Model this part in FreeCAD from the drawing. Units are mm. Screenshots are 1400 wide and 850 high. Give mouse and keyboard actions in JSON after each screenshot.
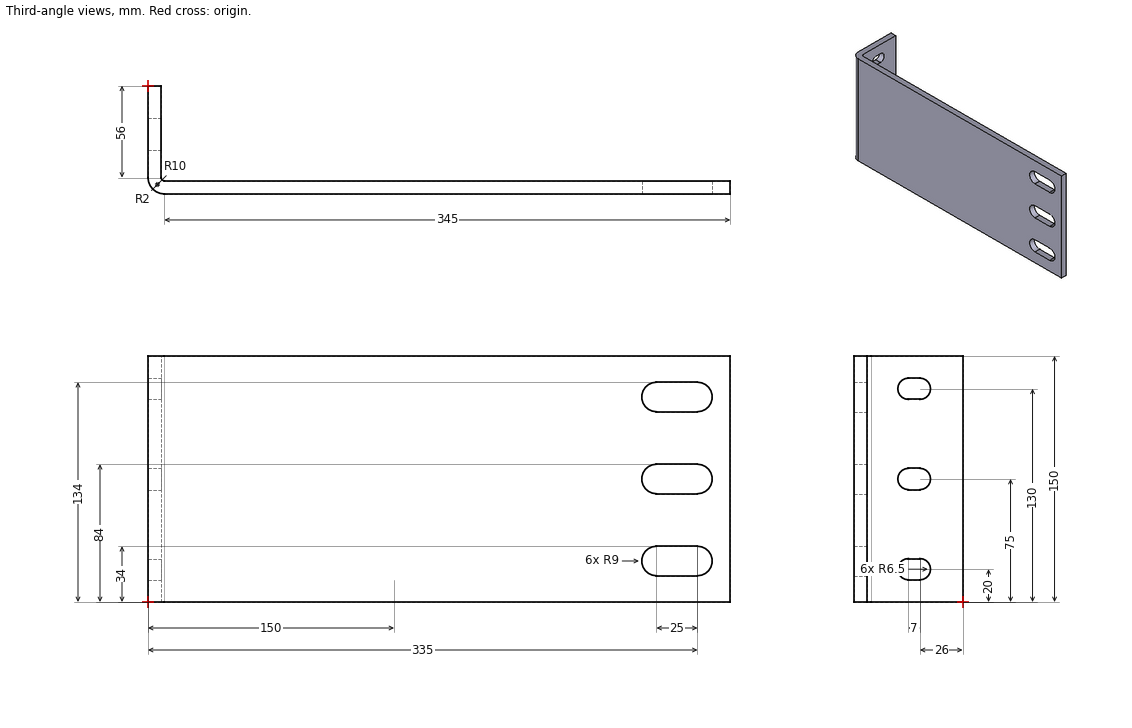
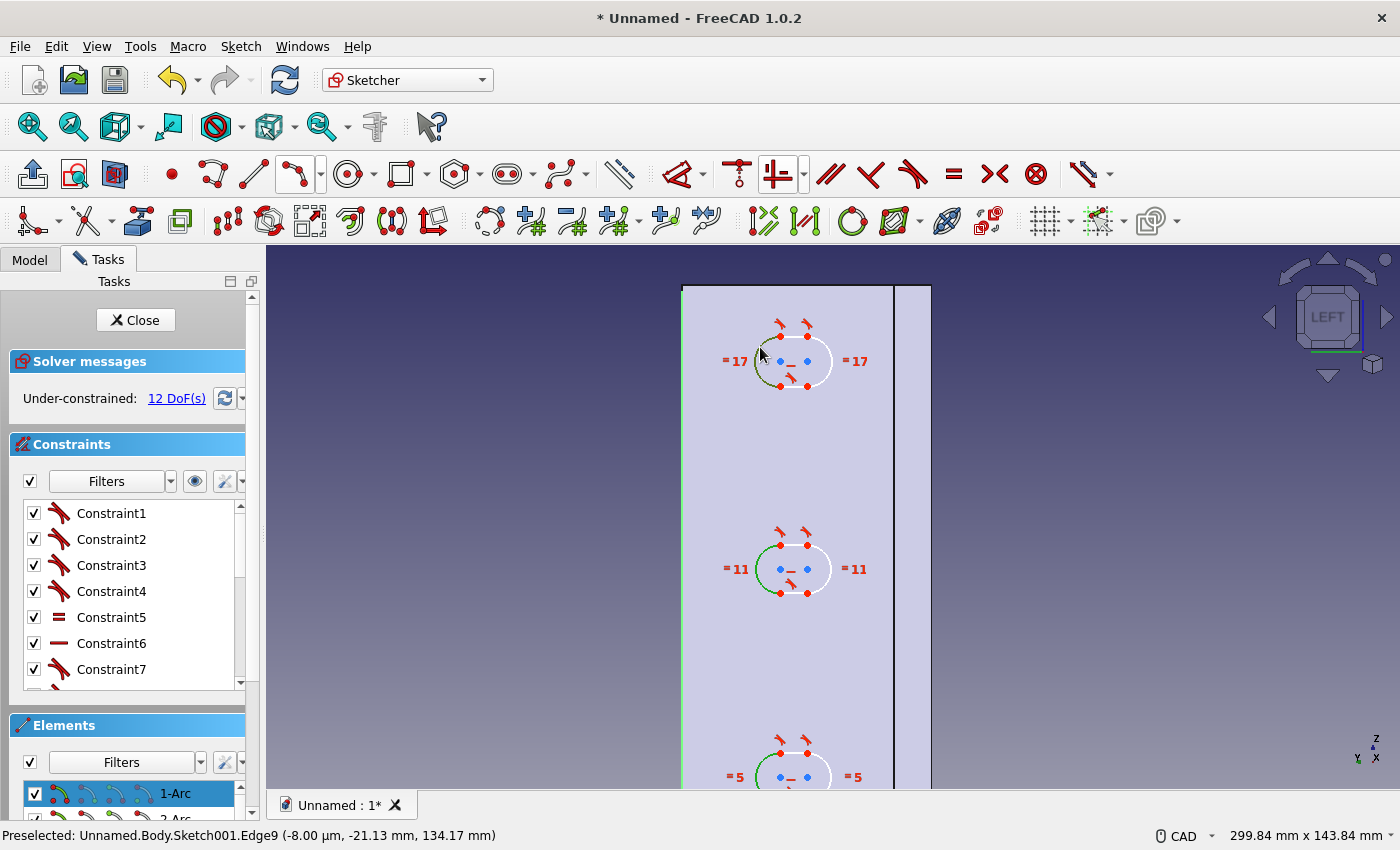
{"action": "left_click", "coordinate": [954, 174]}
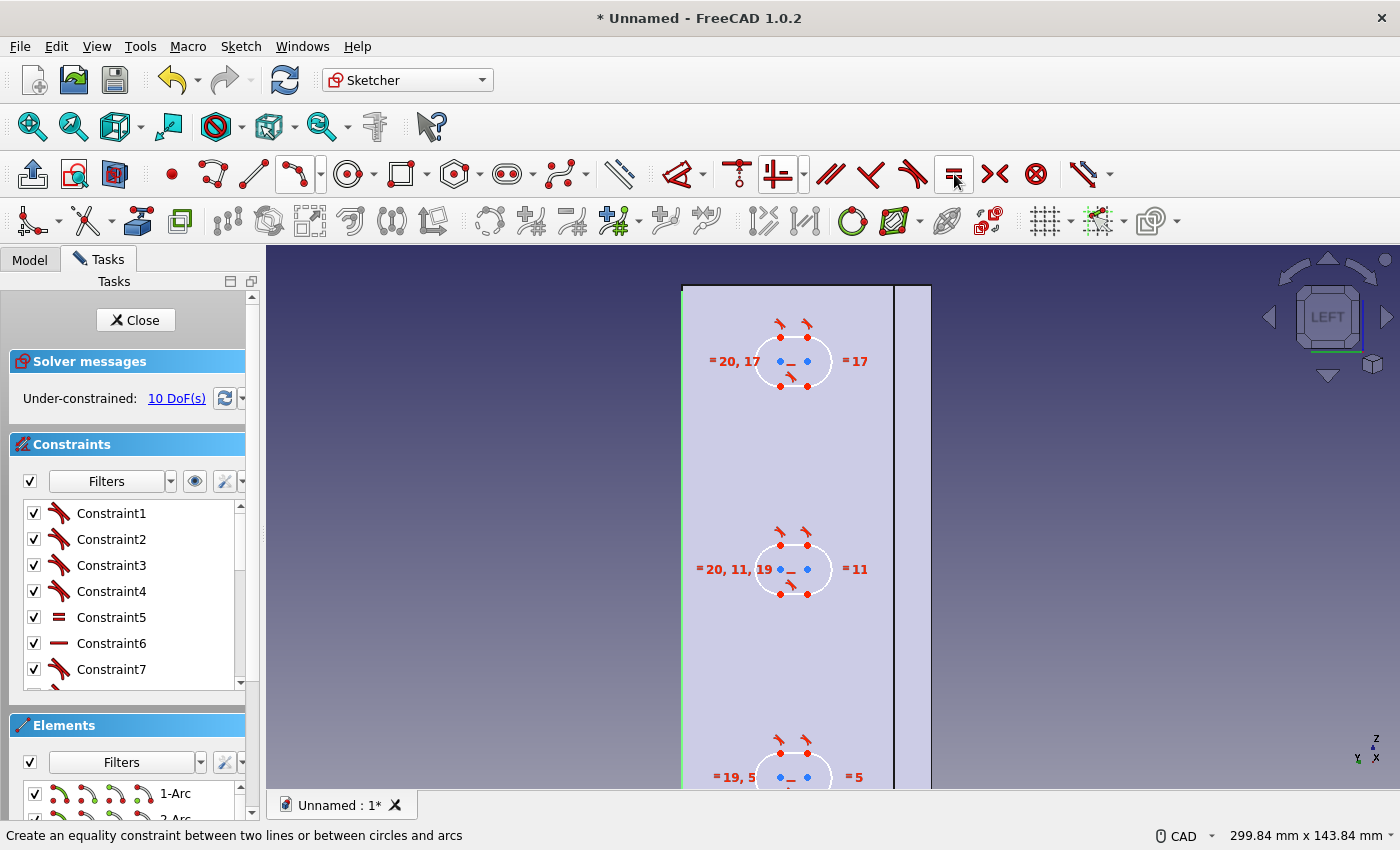
{"action": "left_click", "coordinate": [676, 174]}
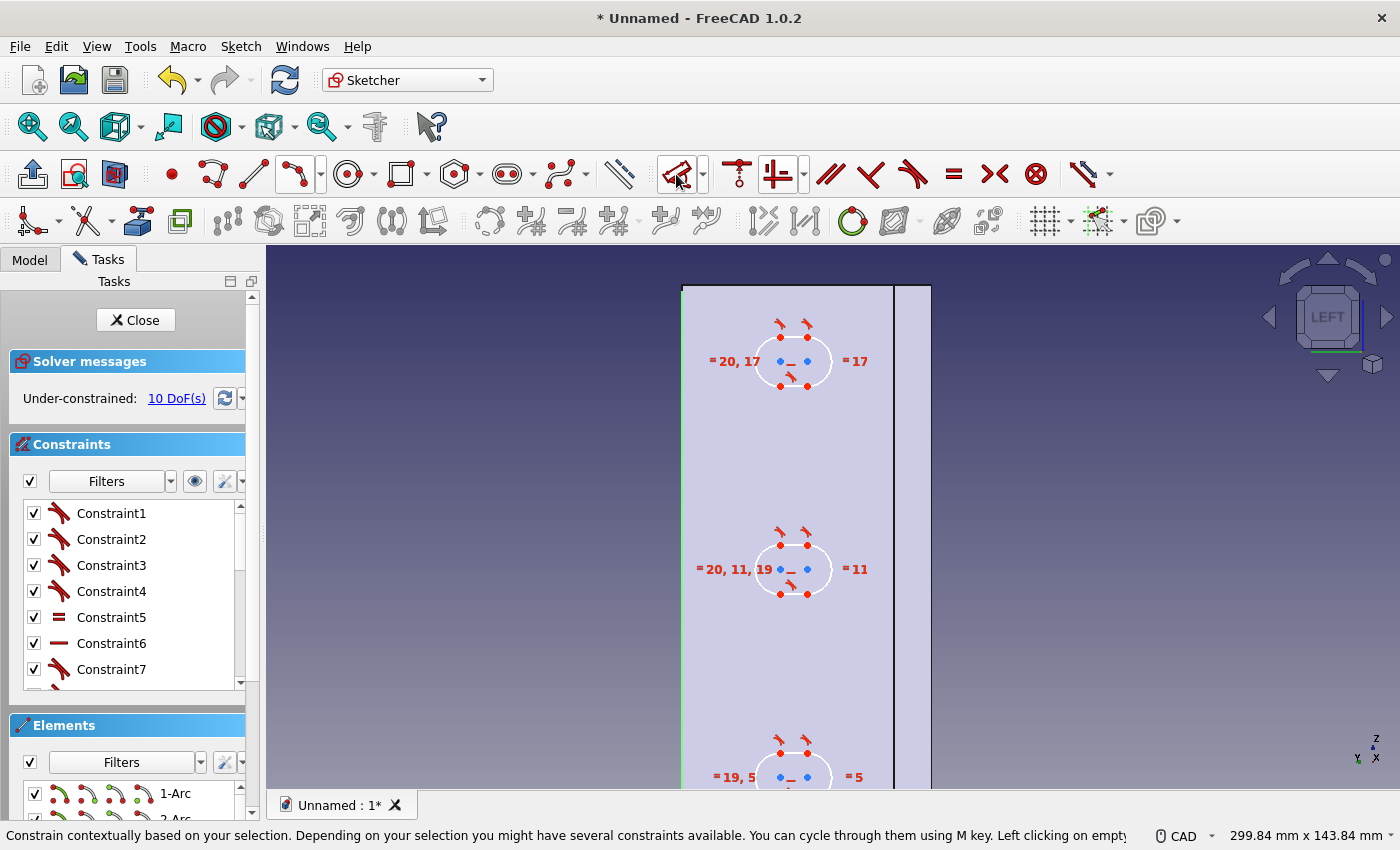
{"action": "scroll", "coordinate": [766, 758], "scroll_direction": "up", "scroll_amount": 3}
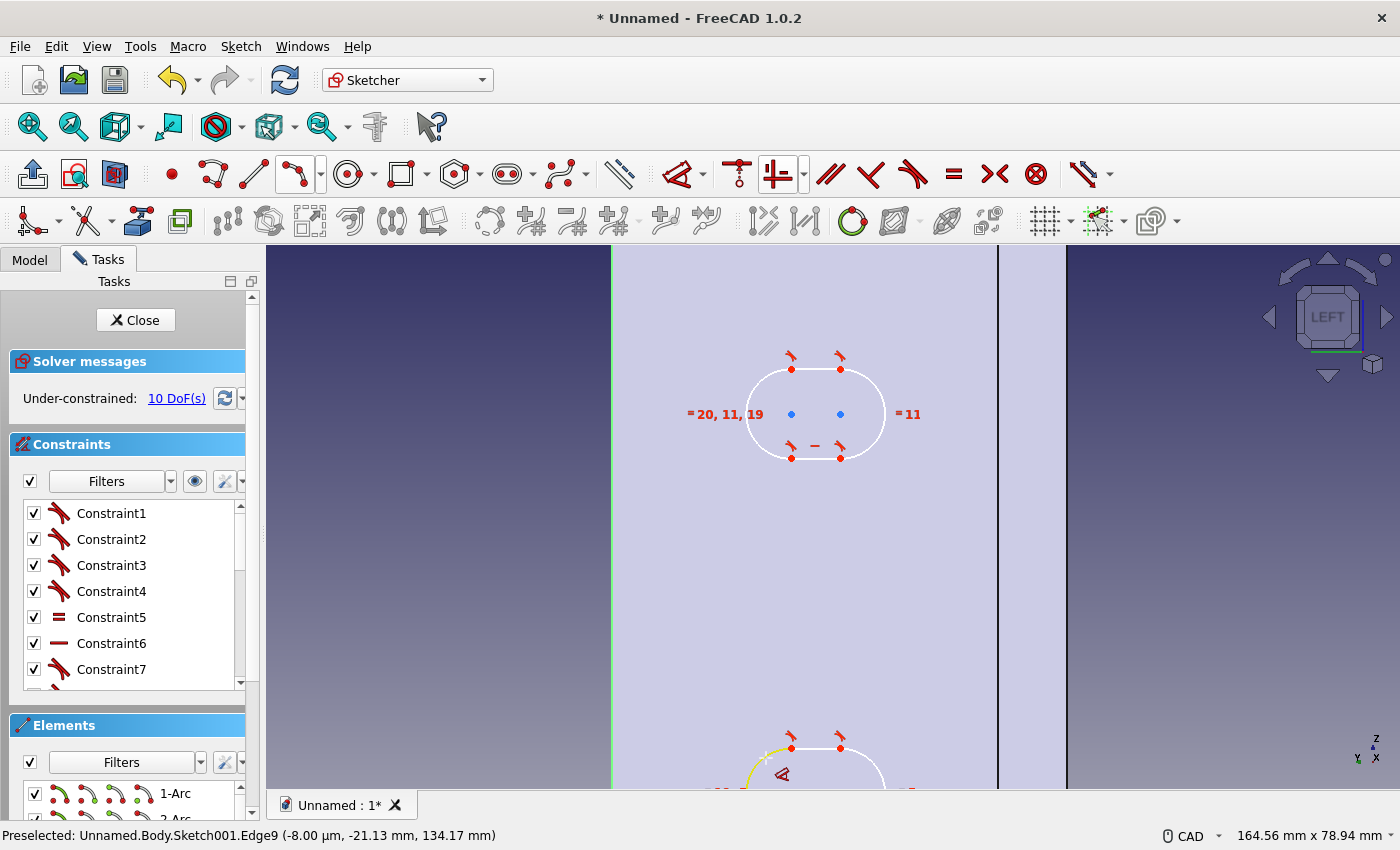
{"action": "left_click", "coordinate": [765, 757]}
{"action": "left_click", "coordinate": [746, 731]}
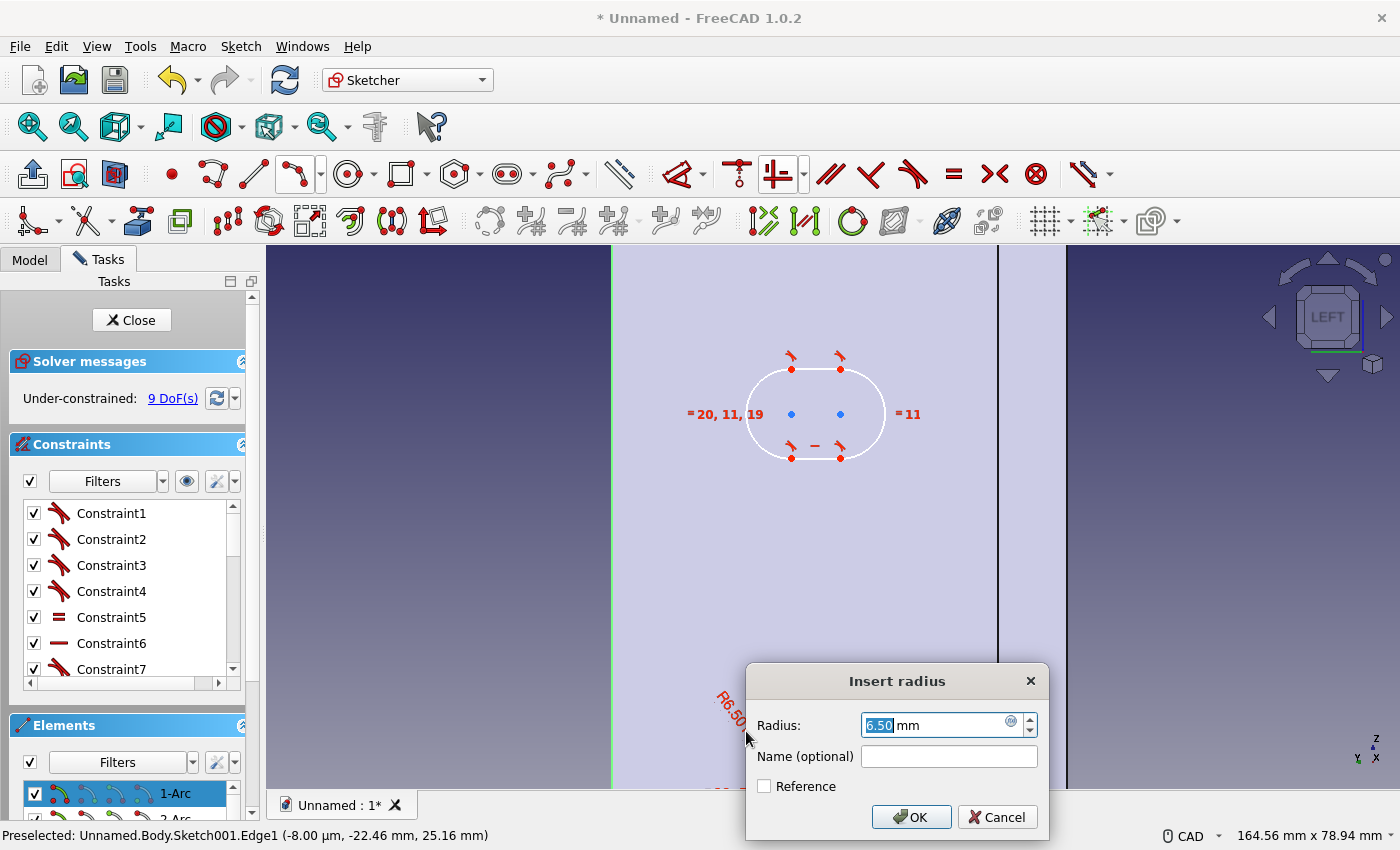
{"action": "type", "text": "6.5"}
{"action": "key", "text": "Return"}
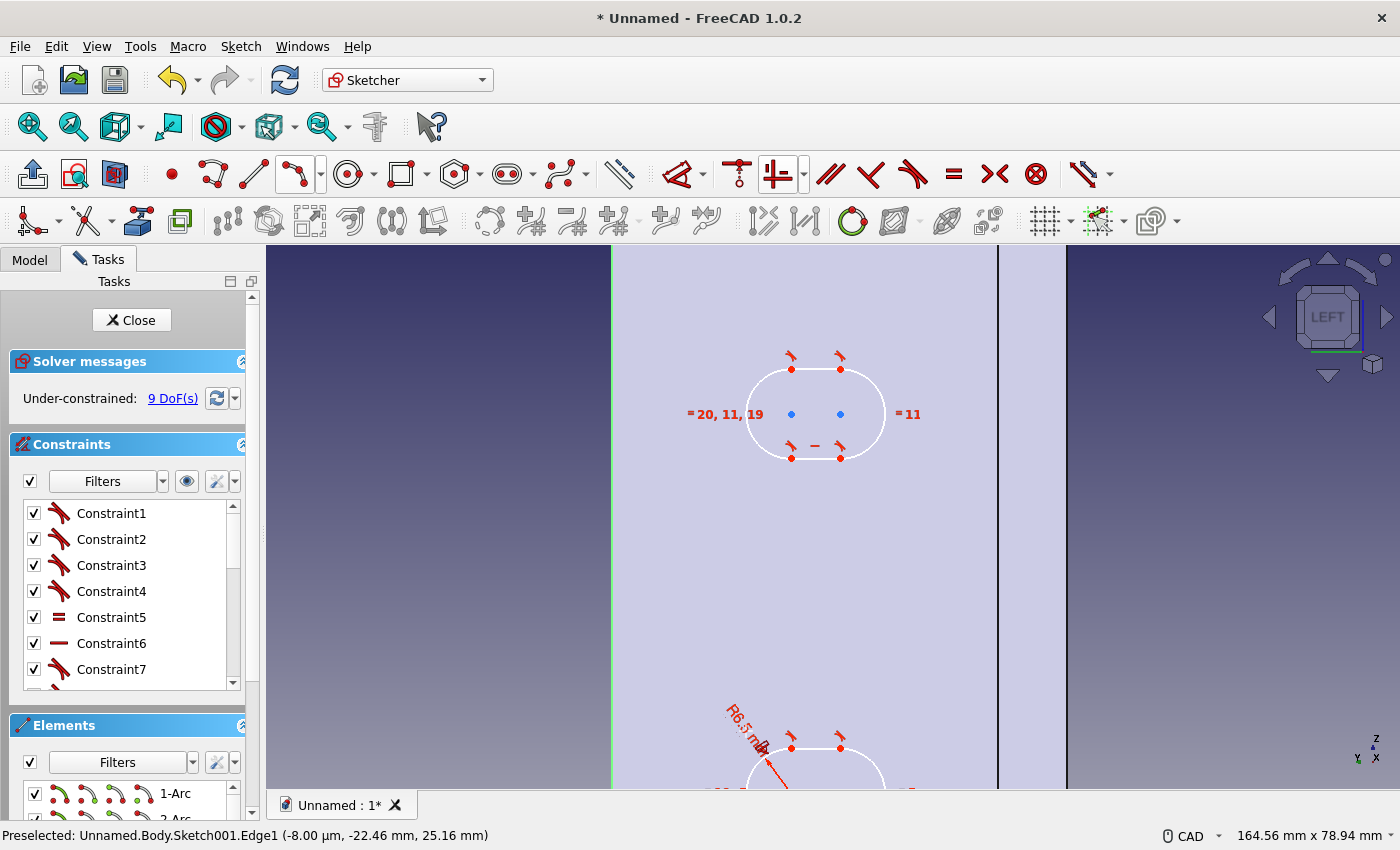
{"action": "left_click", "coordinate": [806, 749]}
{"action": "left_click", "coordinate": [827, 715]}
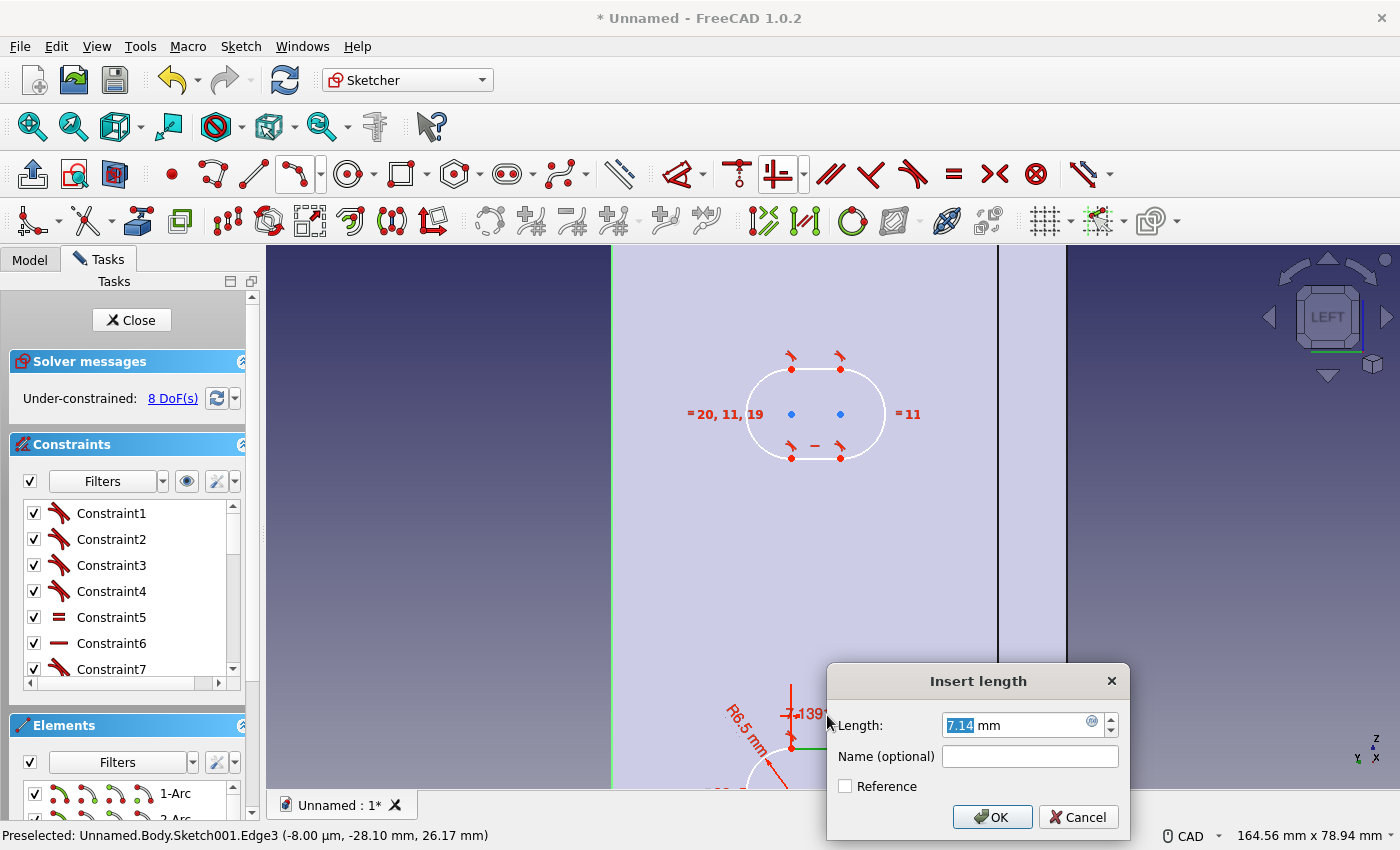
{"action": "type", "text": "7"}
{"action": "key", "text": "Return"}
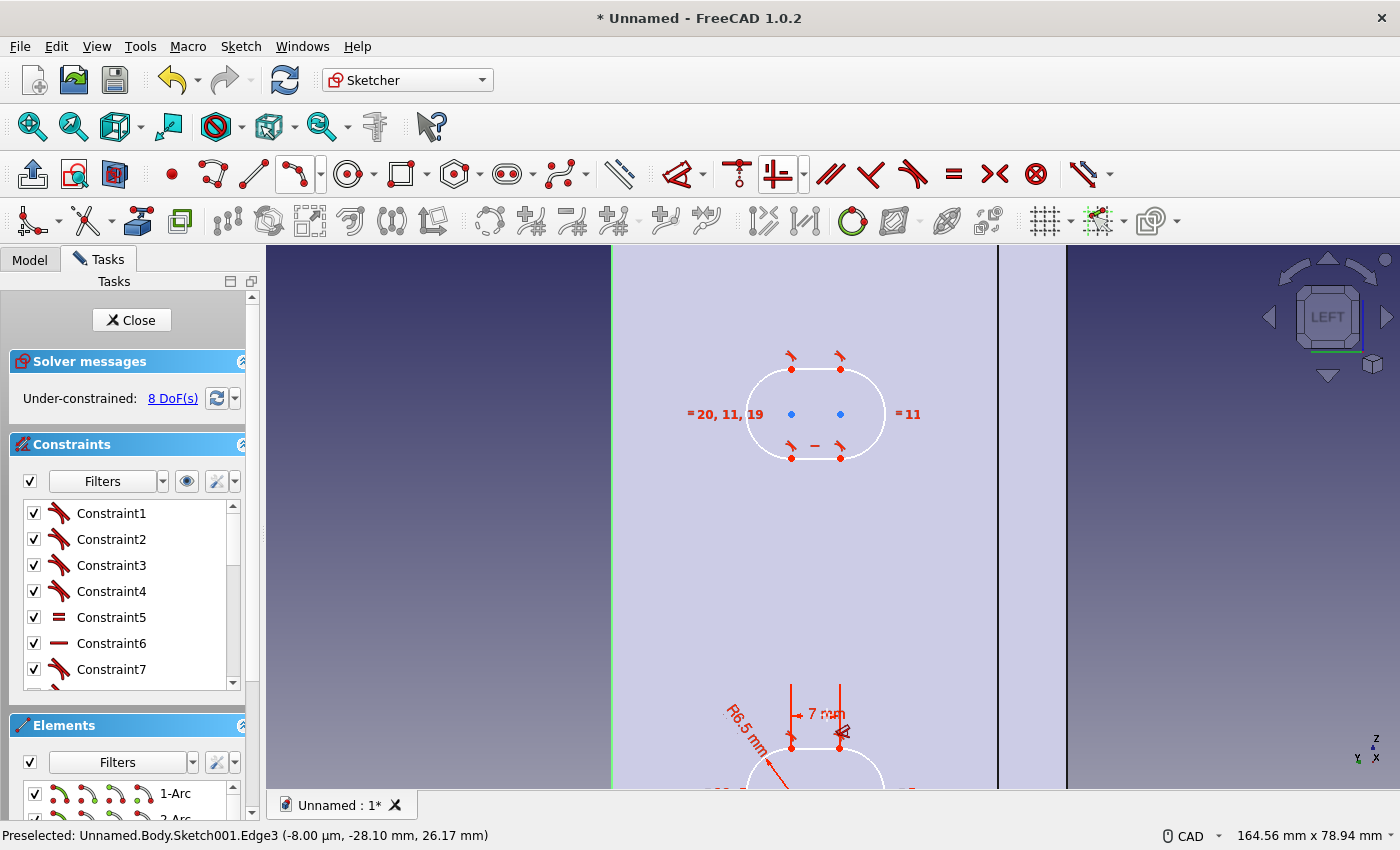
{"action": "left_click", "coordinate": [806, 369]}
{"action": "left_click", "coordinate": [816, 335]}